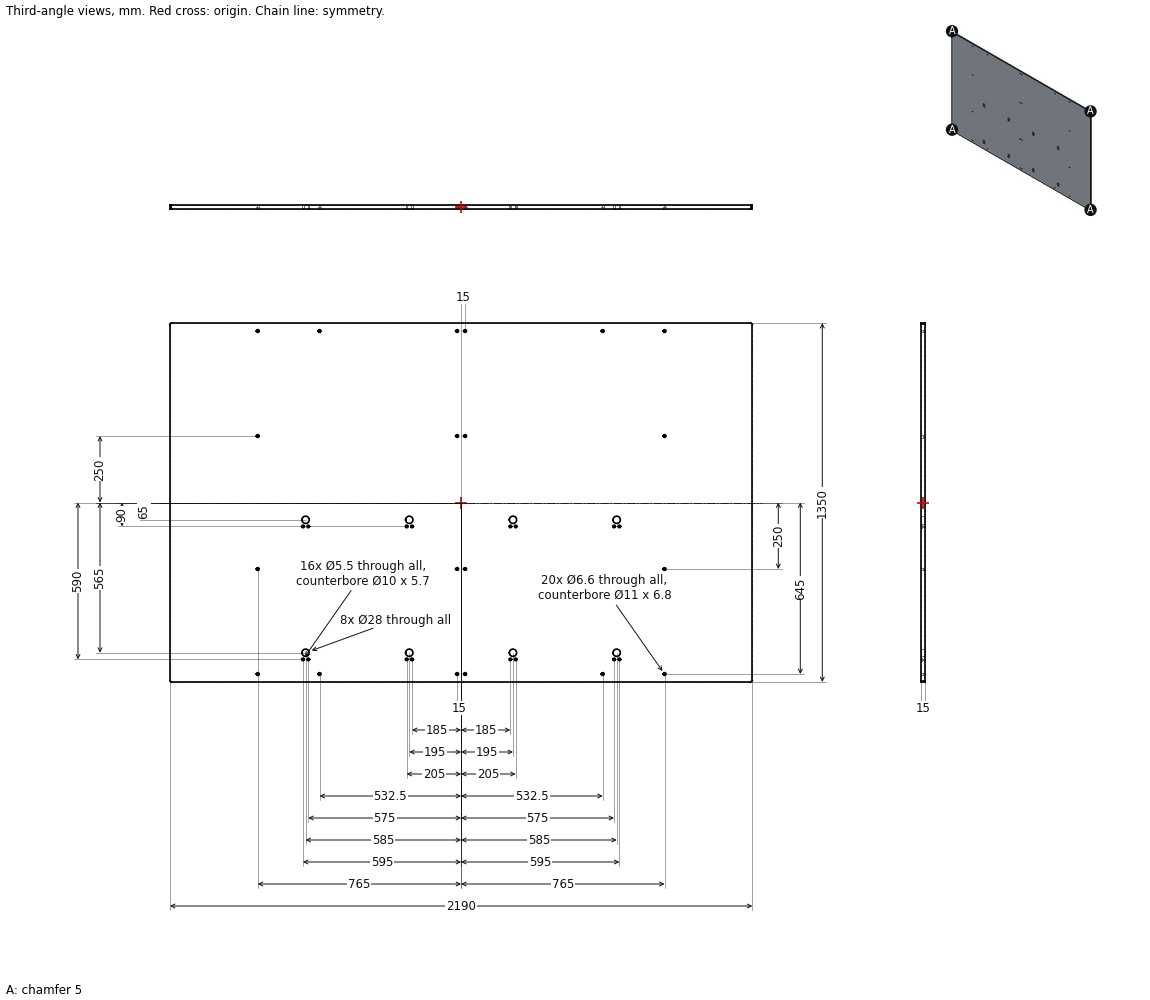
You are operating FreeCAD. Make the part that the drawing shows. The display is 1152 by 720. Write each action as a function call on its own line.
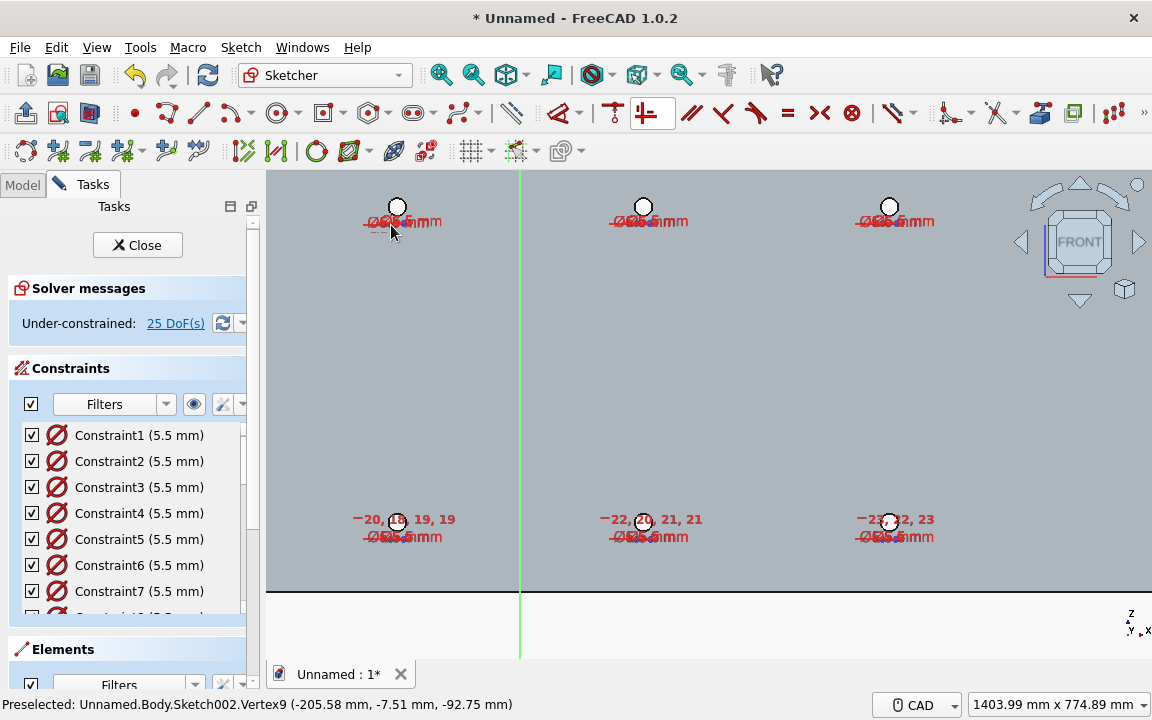
key(v)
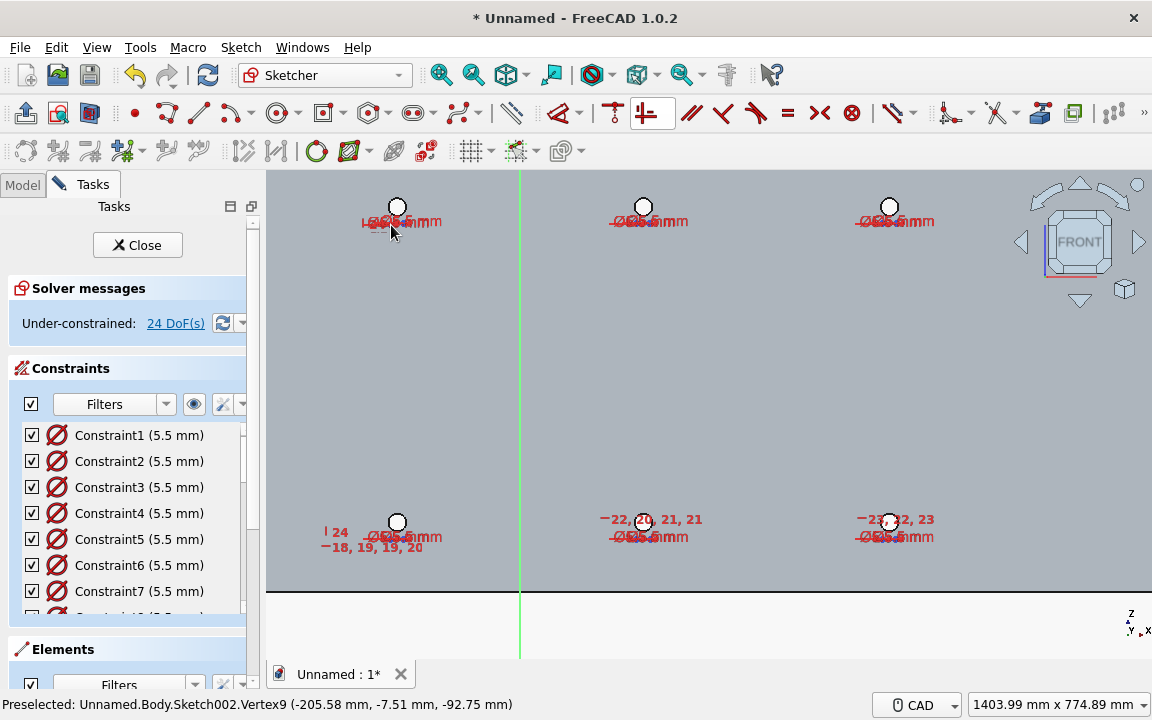
click(404, 539)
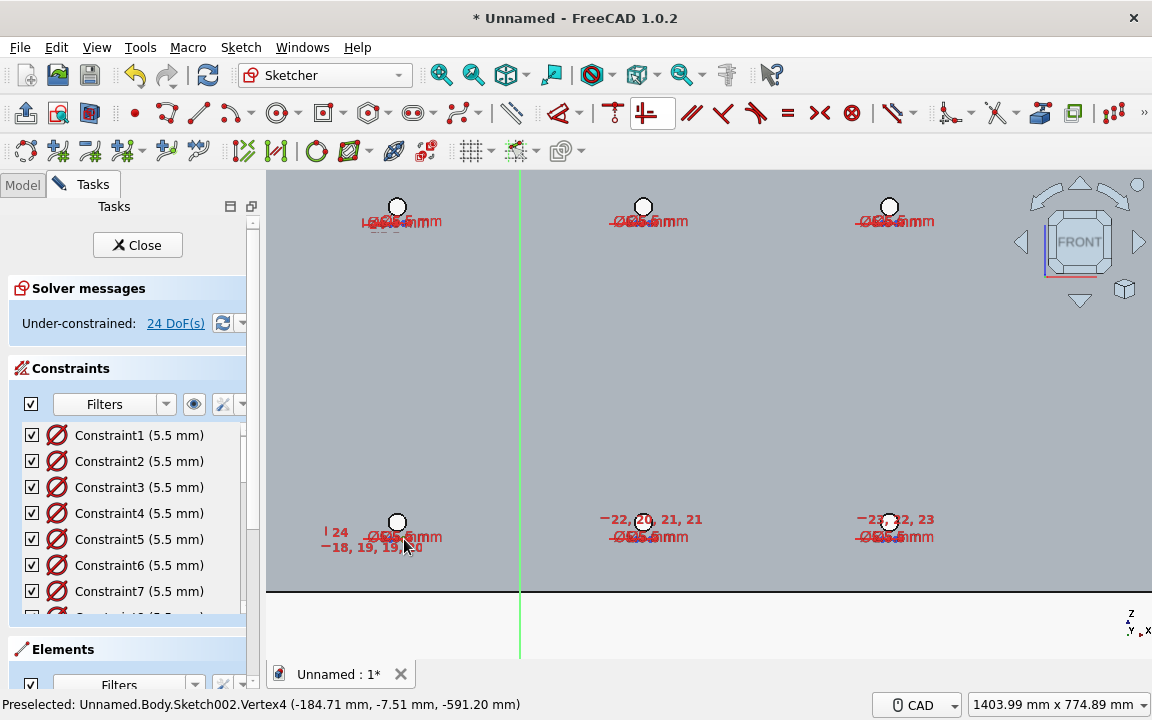
click(404, 223)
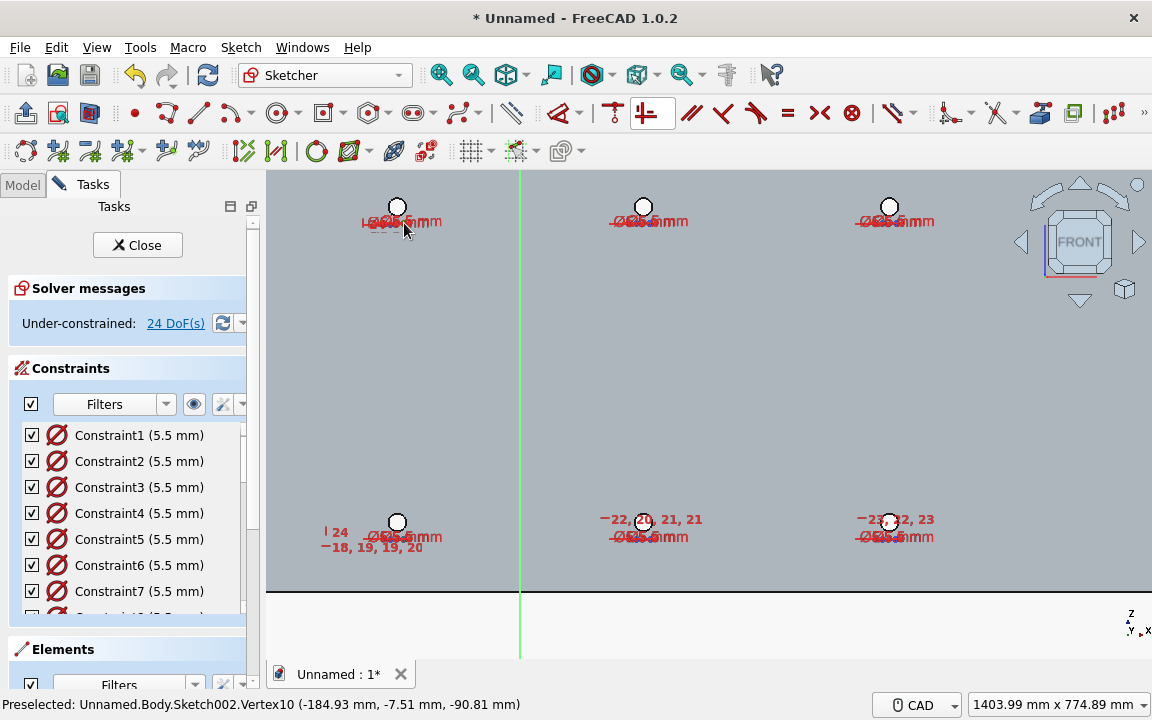
key(v)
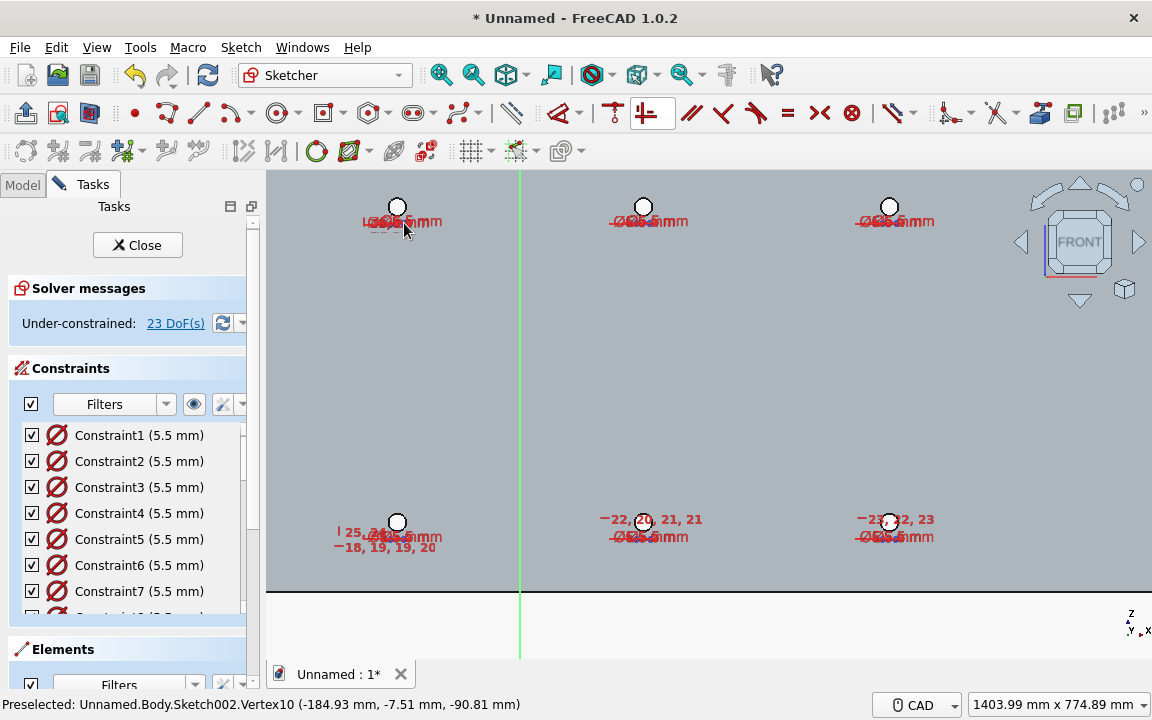
scroll(391, 225, up, 4)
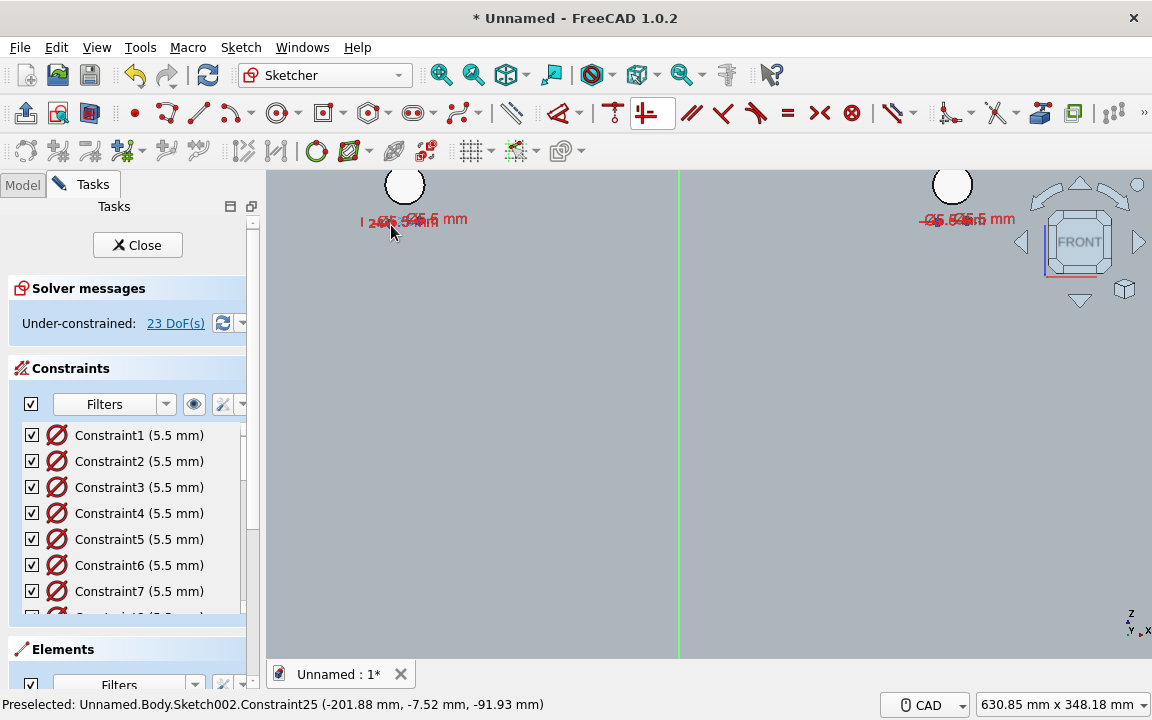
scroll(390, 224, up, 4)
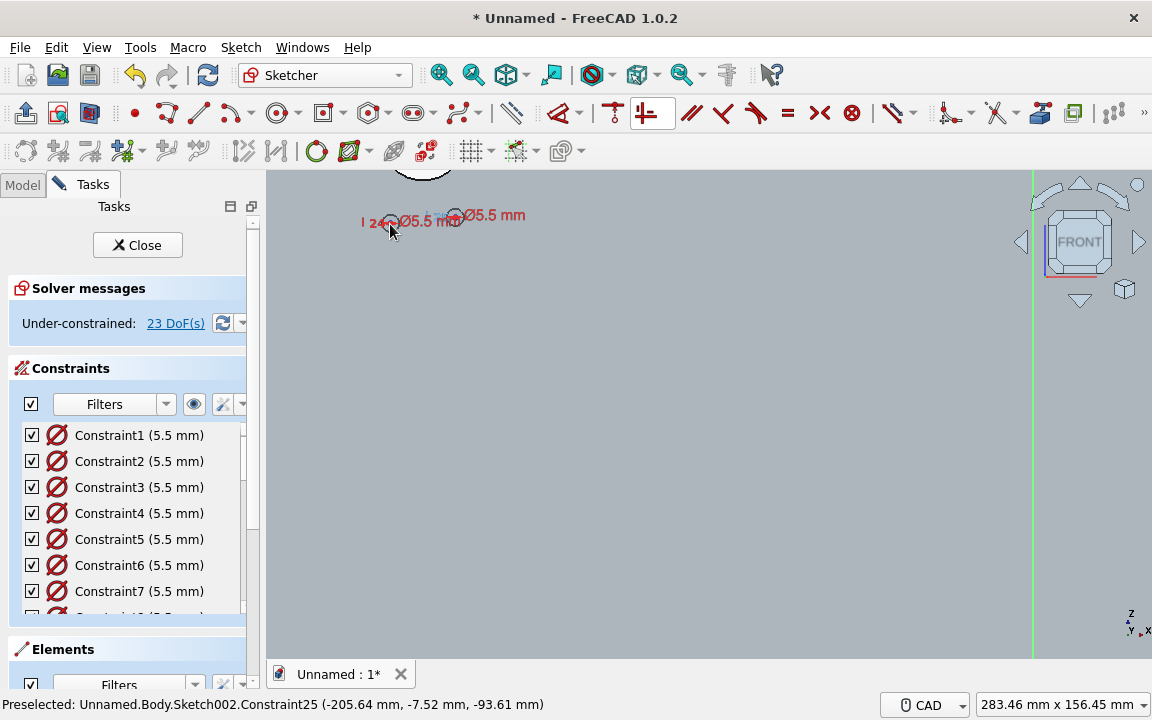
click(391, 223)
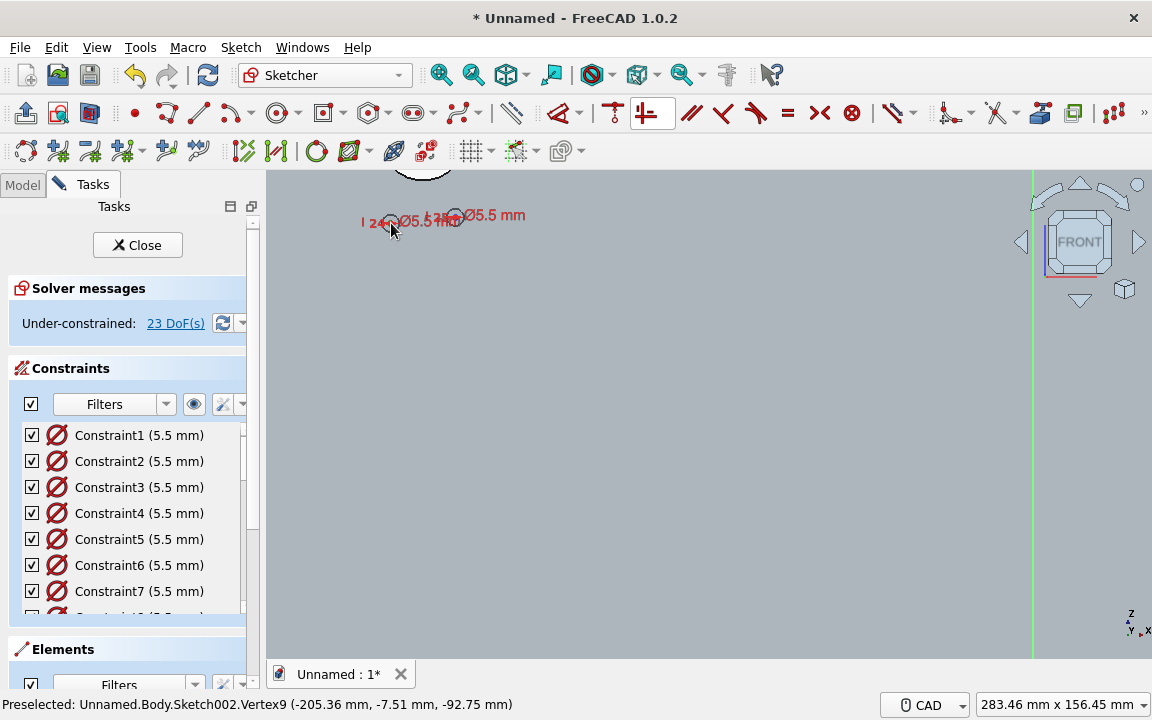
scroll(579, 345, down, 10)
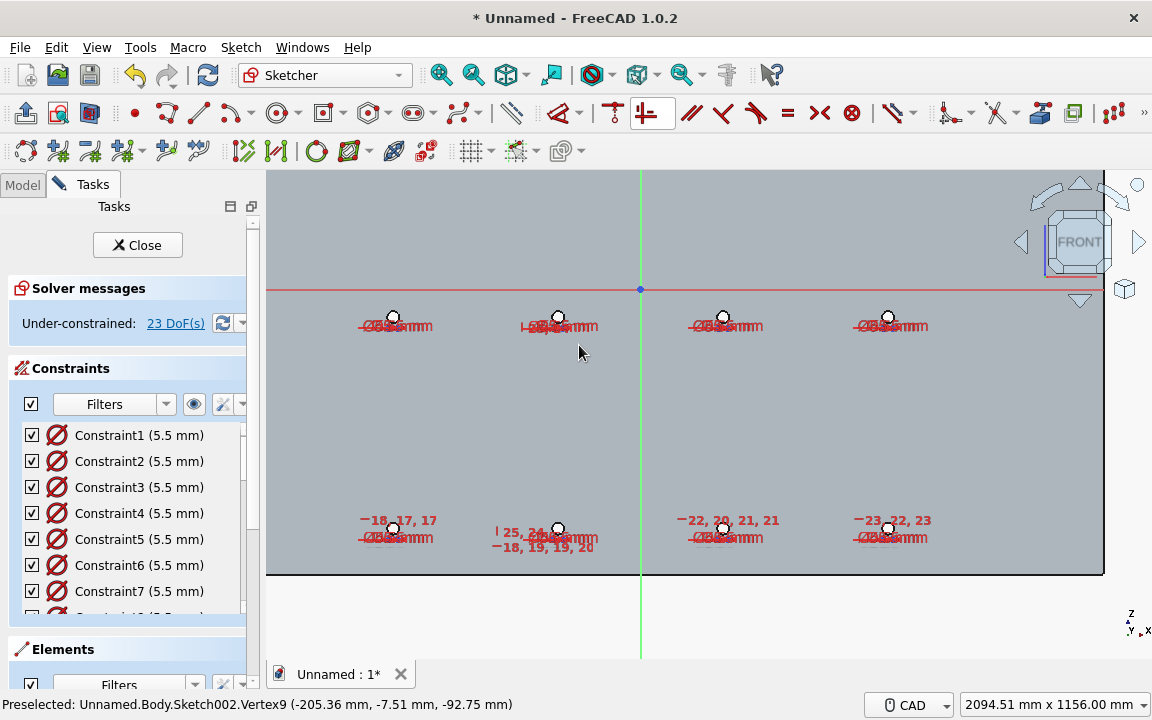
scroll(563, 328, up, 2)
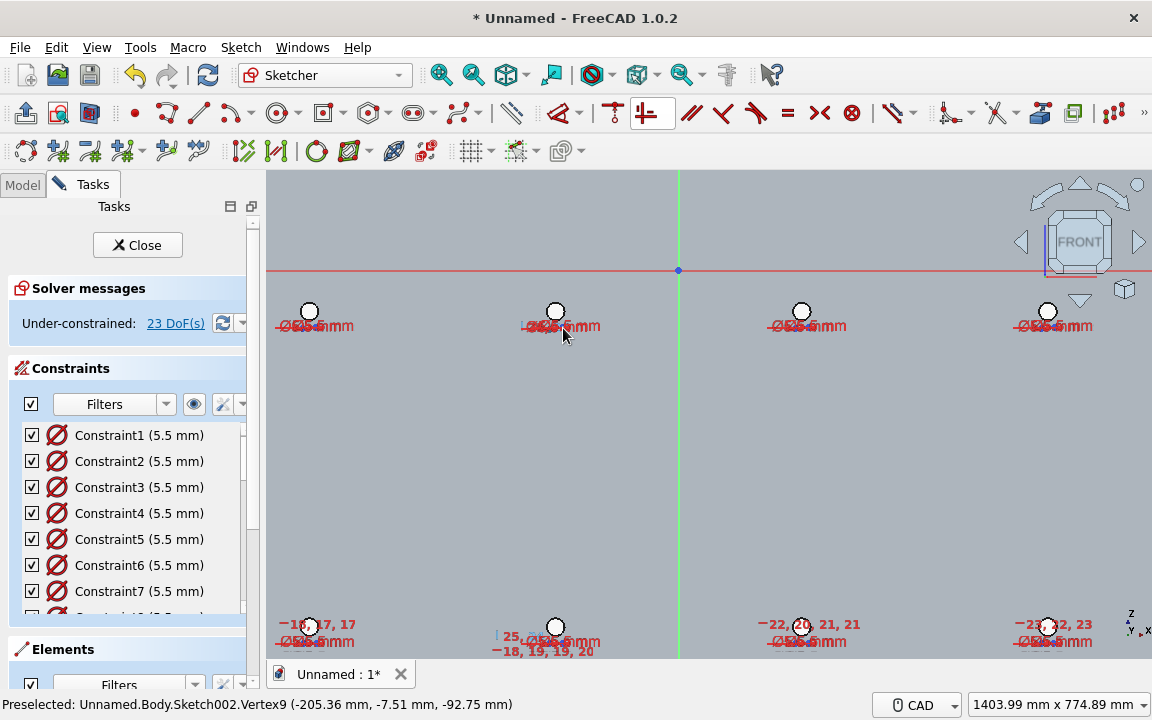
scroll(562, 328, up, 4)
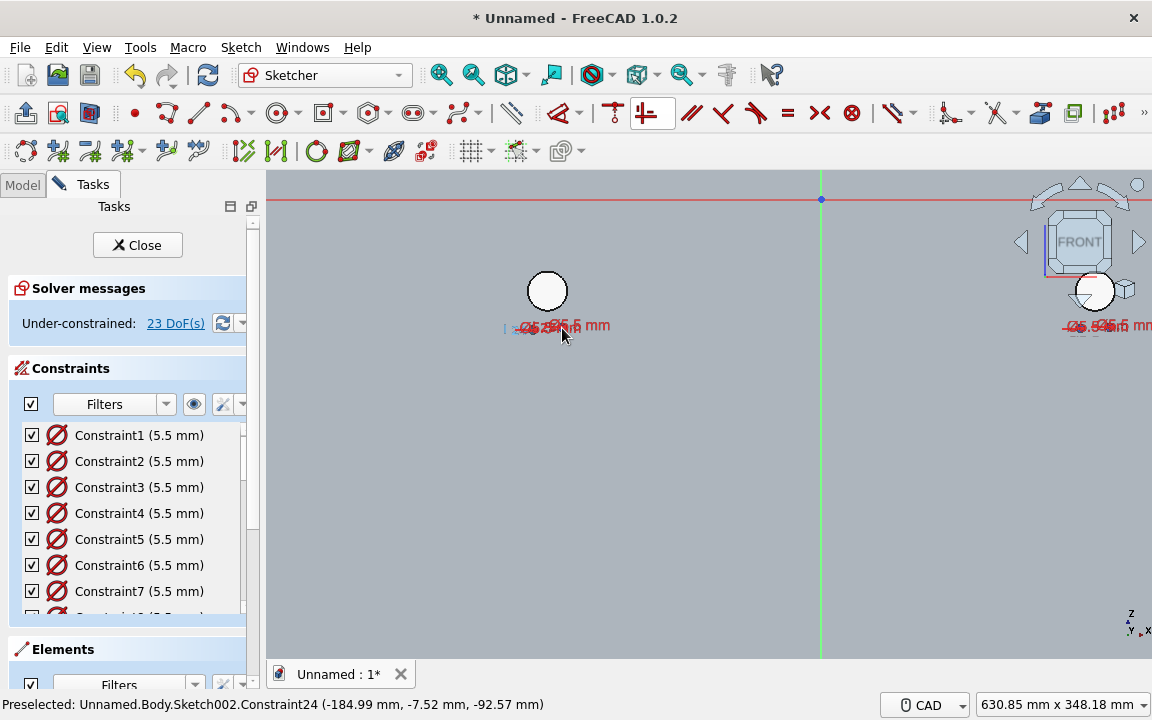
click(562, 327)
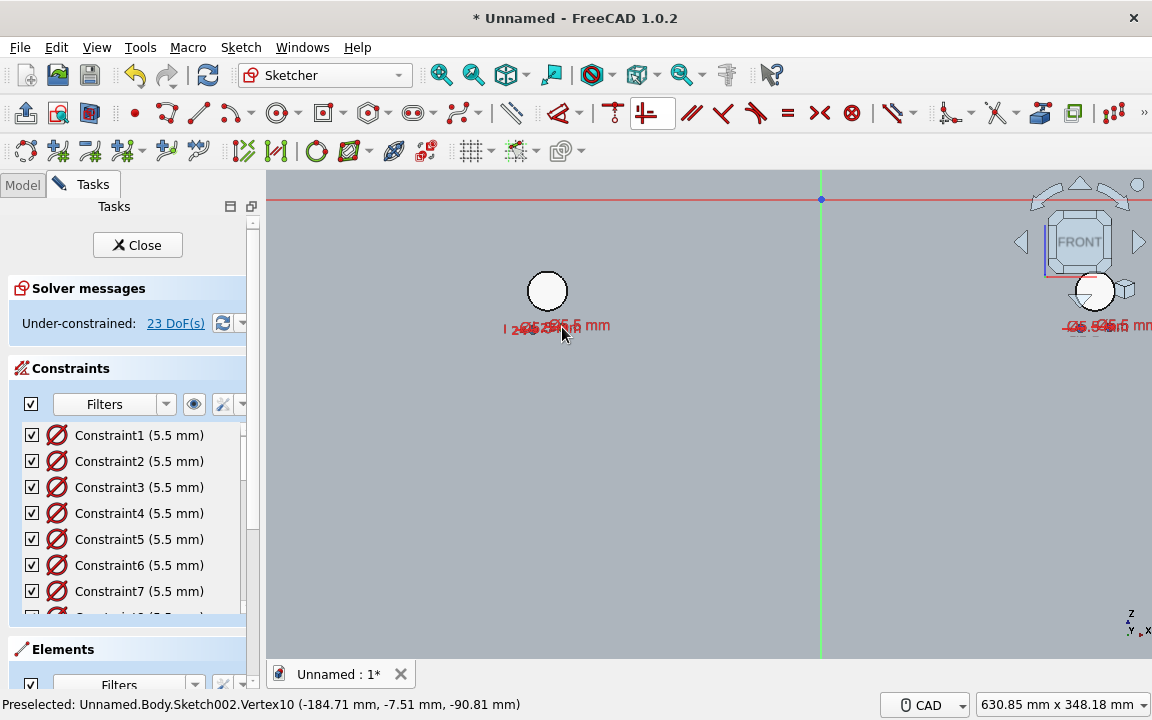
key(h)